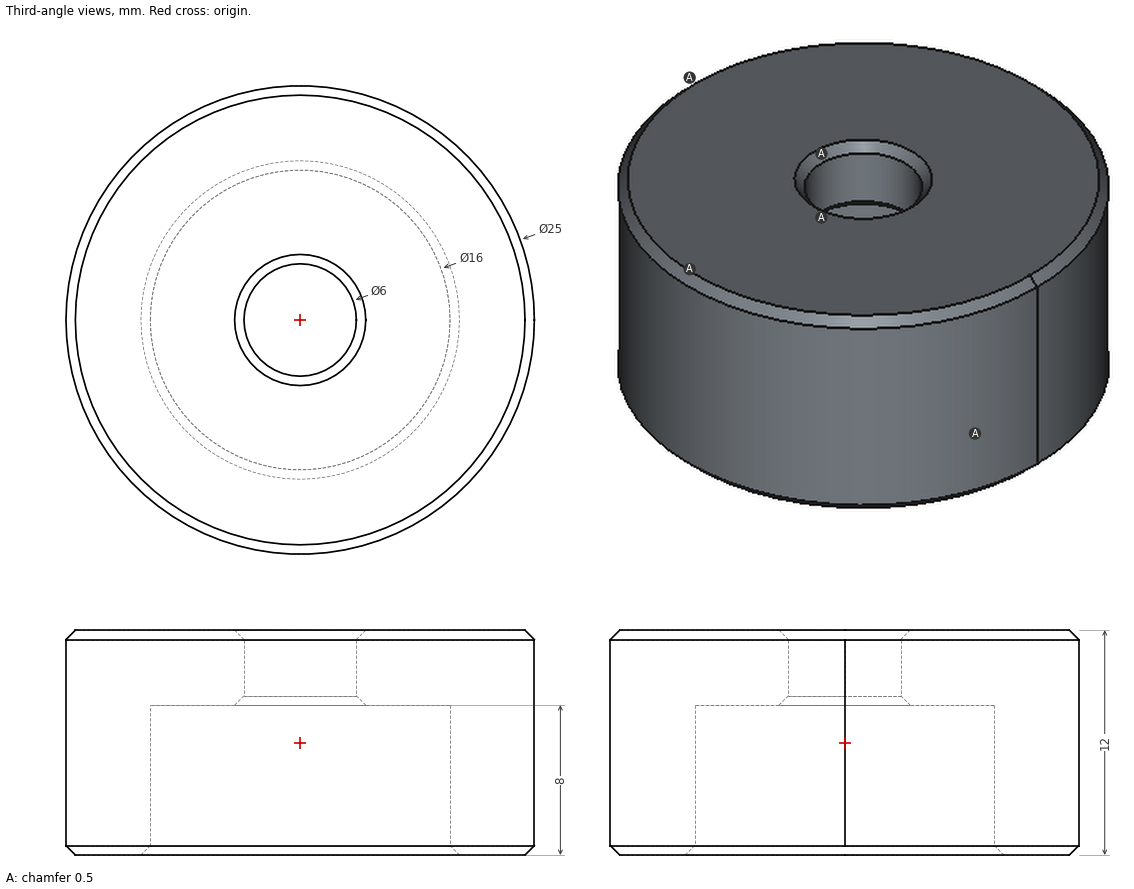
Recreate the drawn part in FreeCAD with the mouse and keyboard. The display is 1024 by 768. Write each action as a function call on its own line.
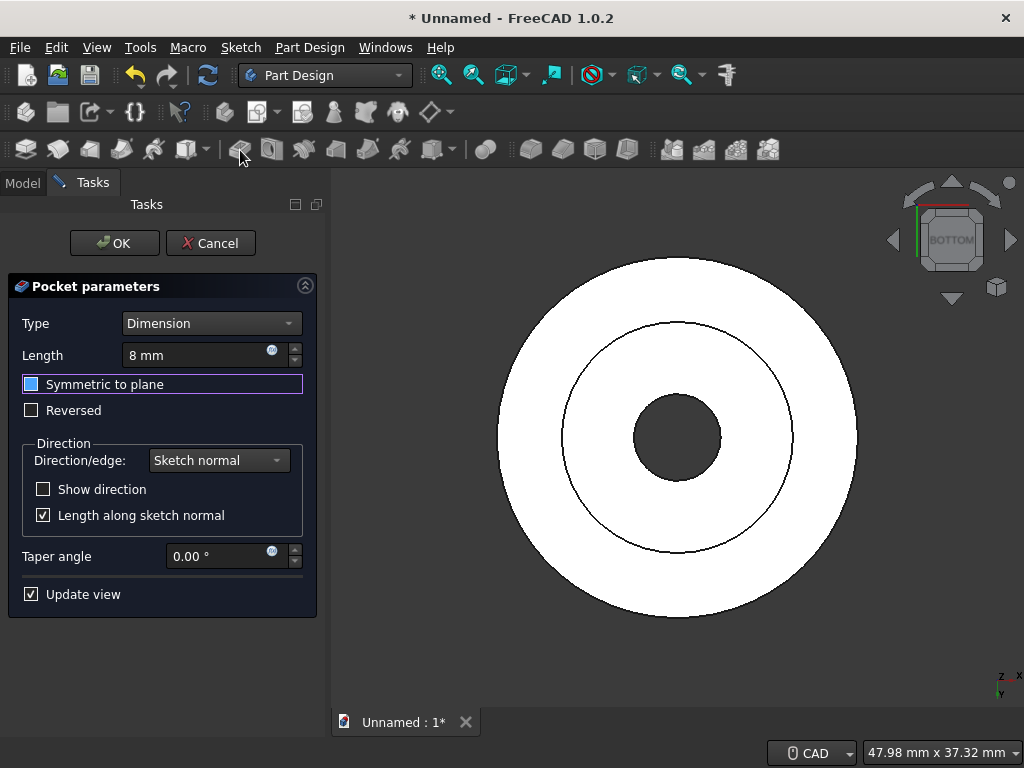
click(115, 243)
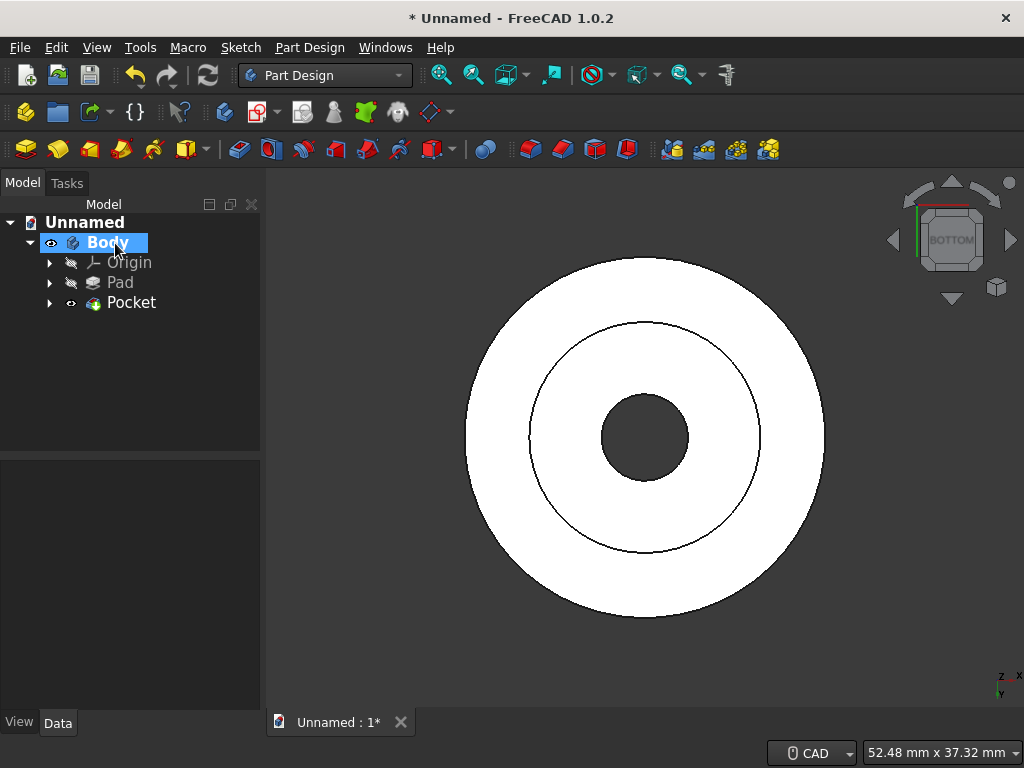
click(602, 437)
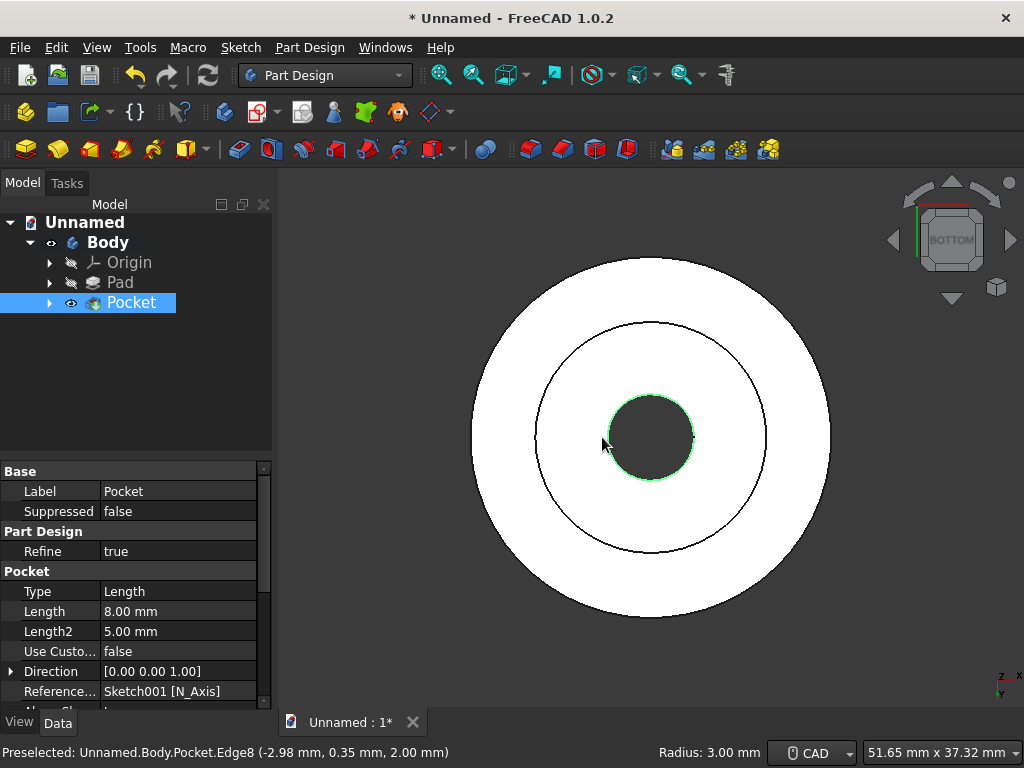
click(557, 369, ctrl)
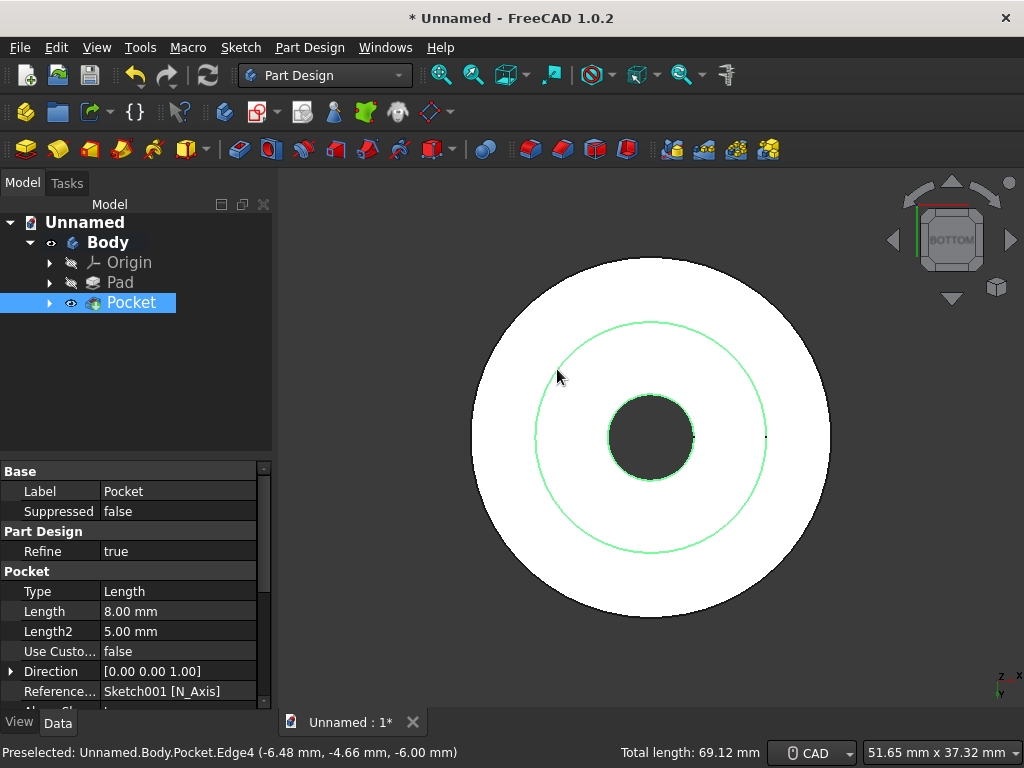
click(470, 437, ctrl)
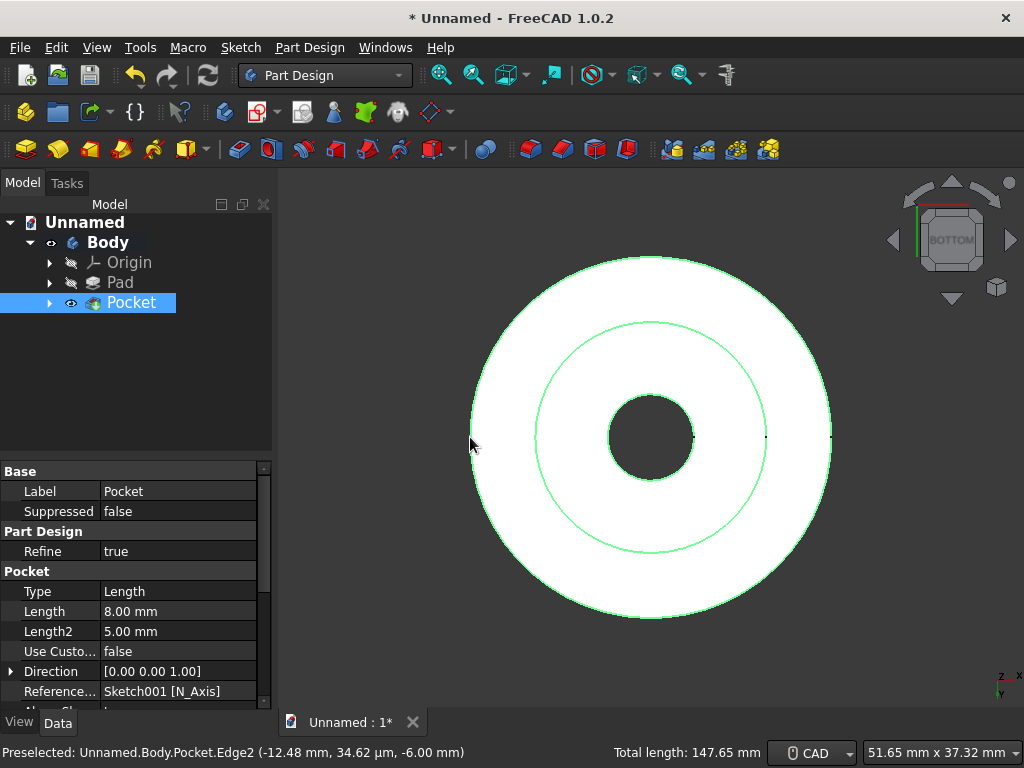
key(0)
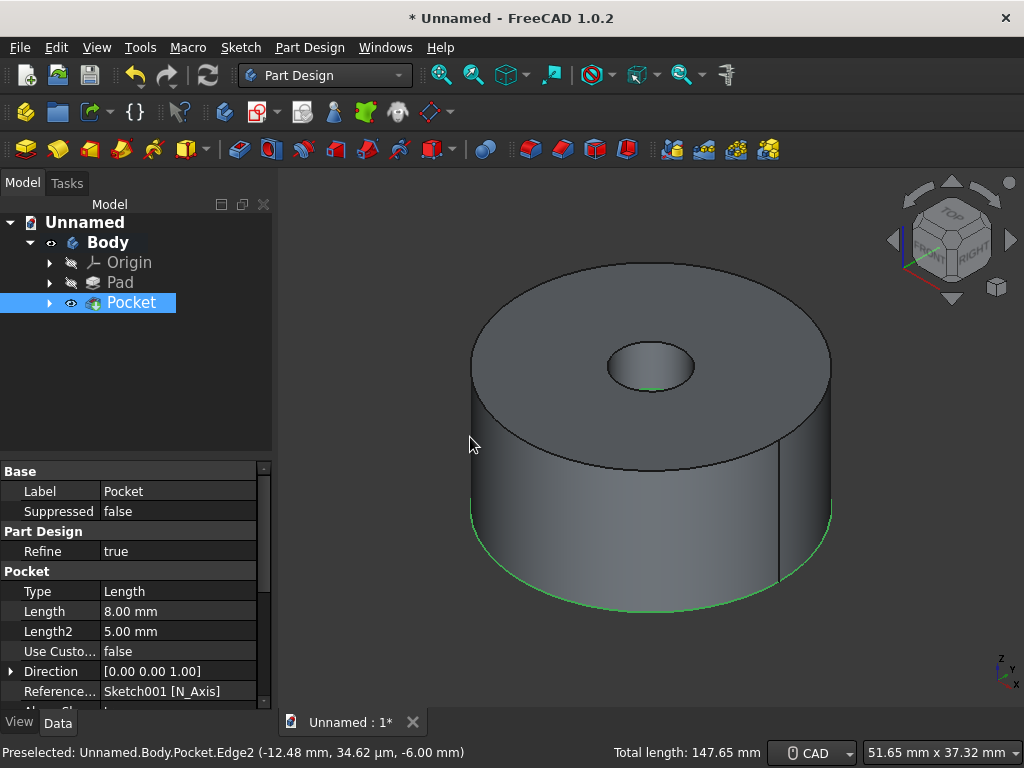
click(490, 413, ctrl)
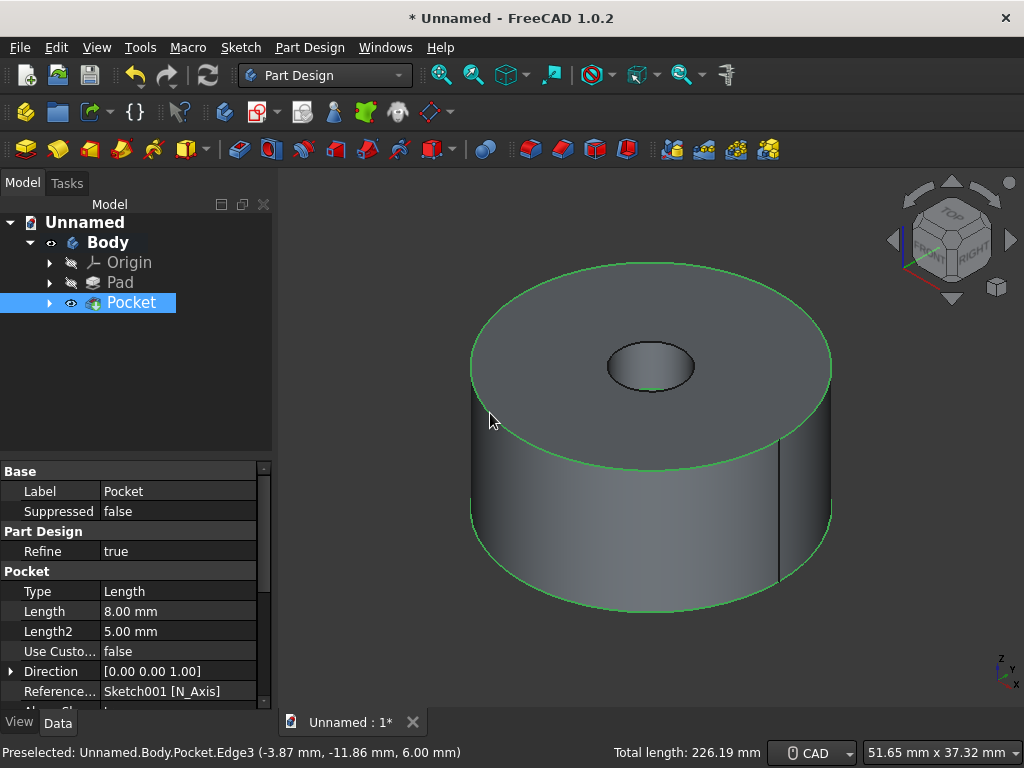
click(620, 348, ctrl)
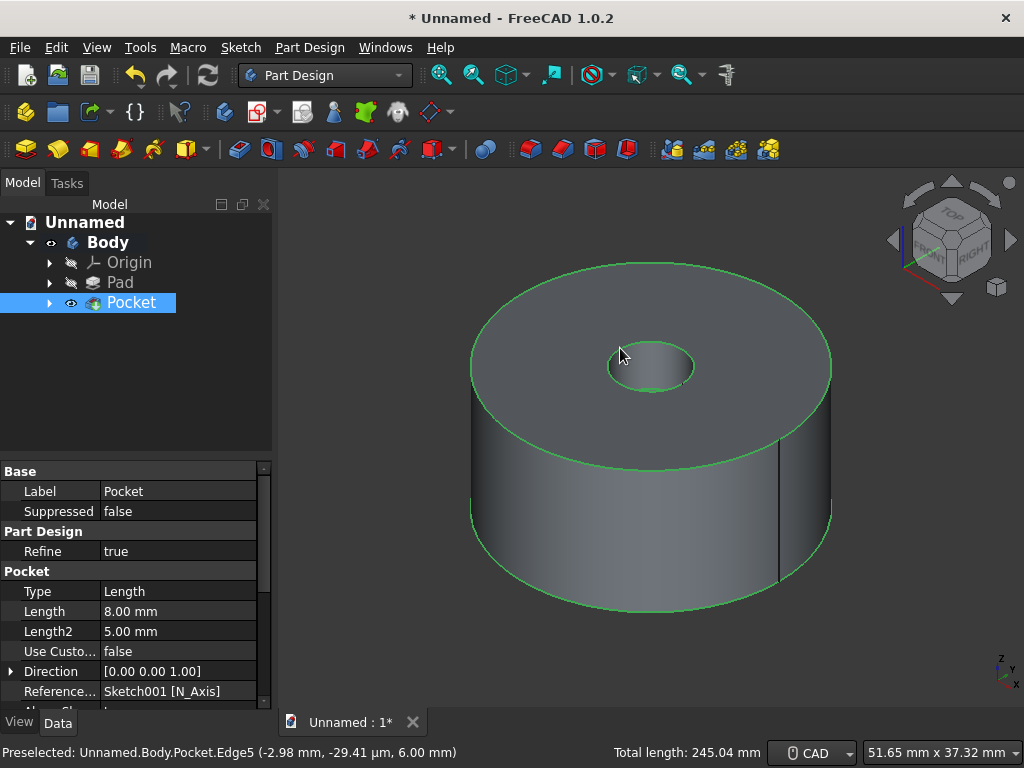
click(564, 150)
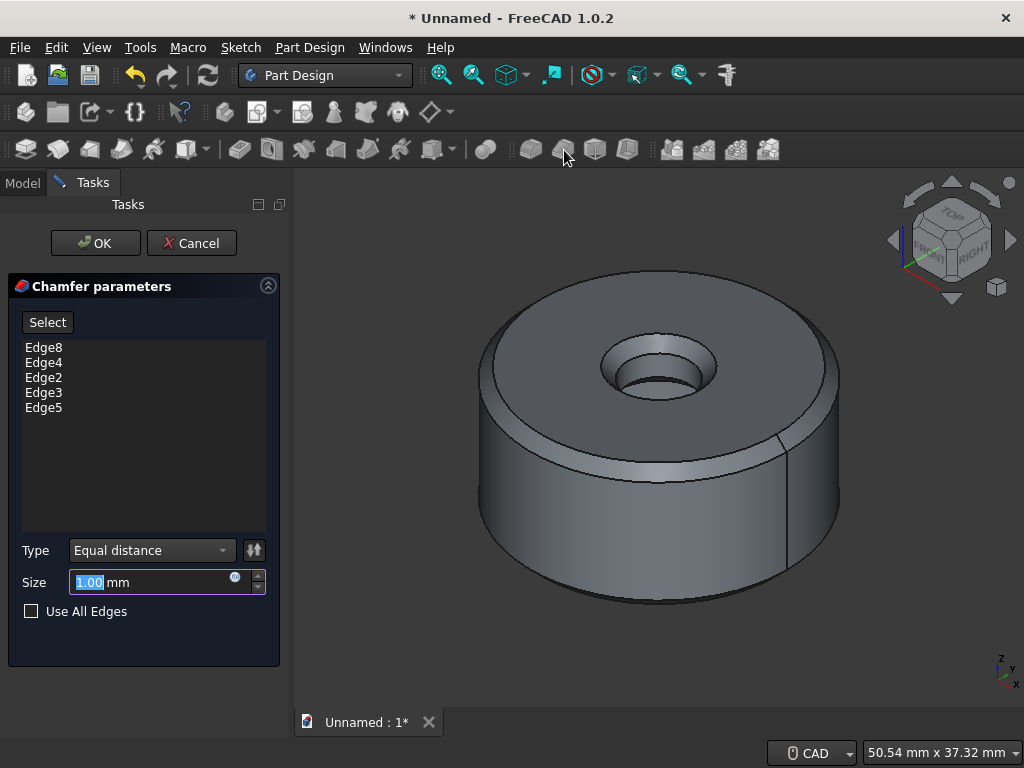
text(0.5)
key(Tab)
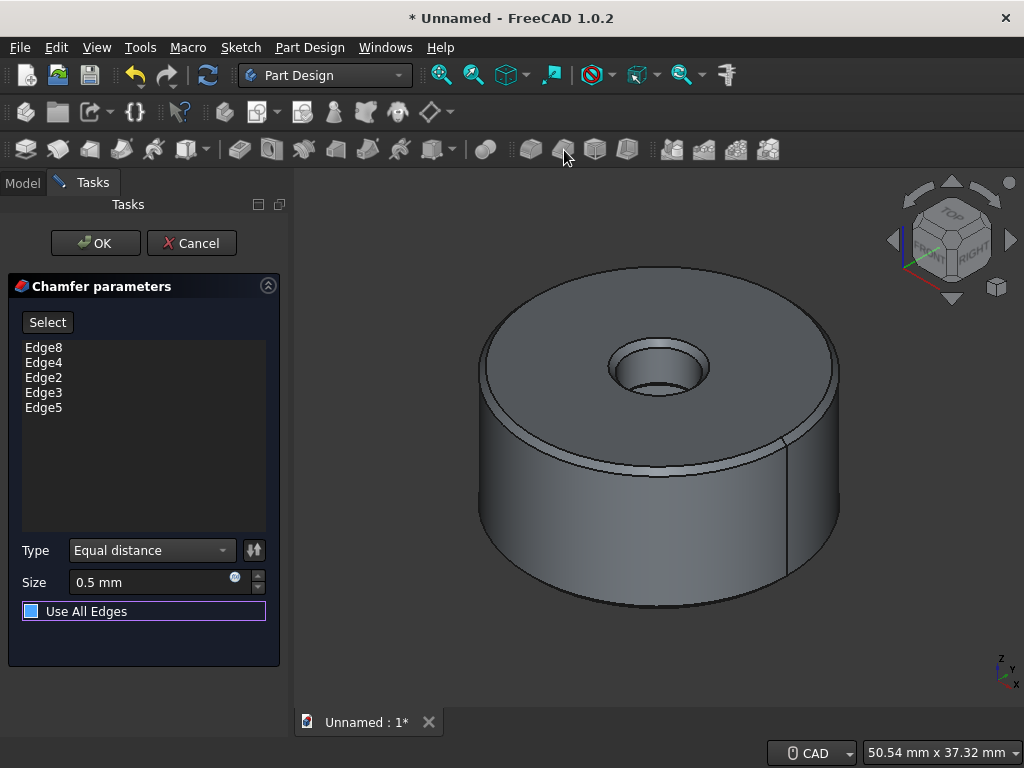
click(96, 243)